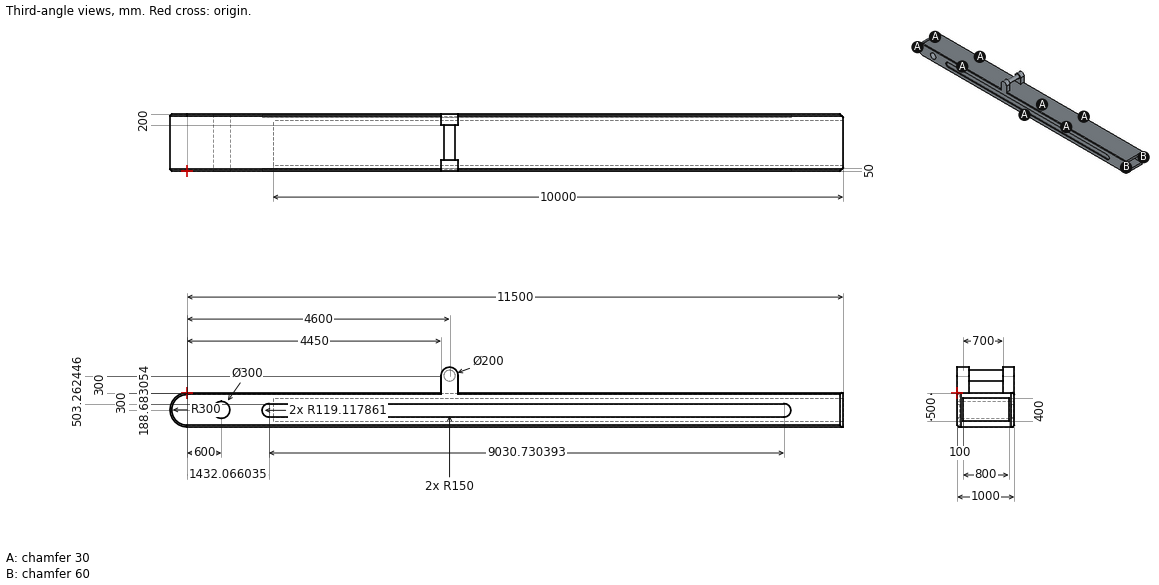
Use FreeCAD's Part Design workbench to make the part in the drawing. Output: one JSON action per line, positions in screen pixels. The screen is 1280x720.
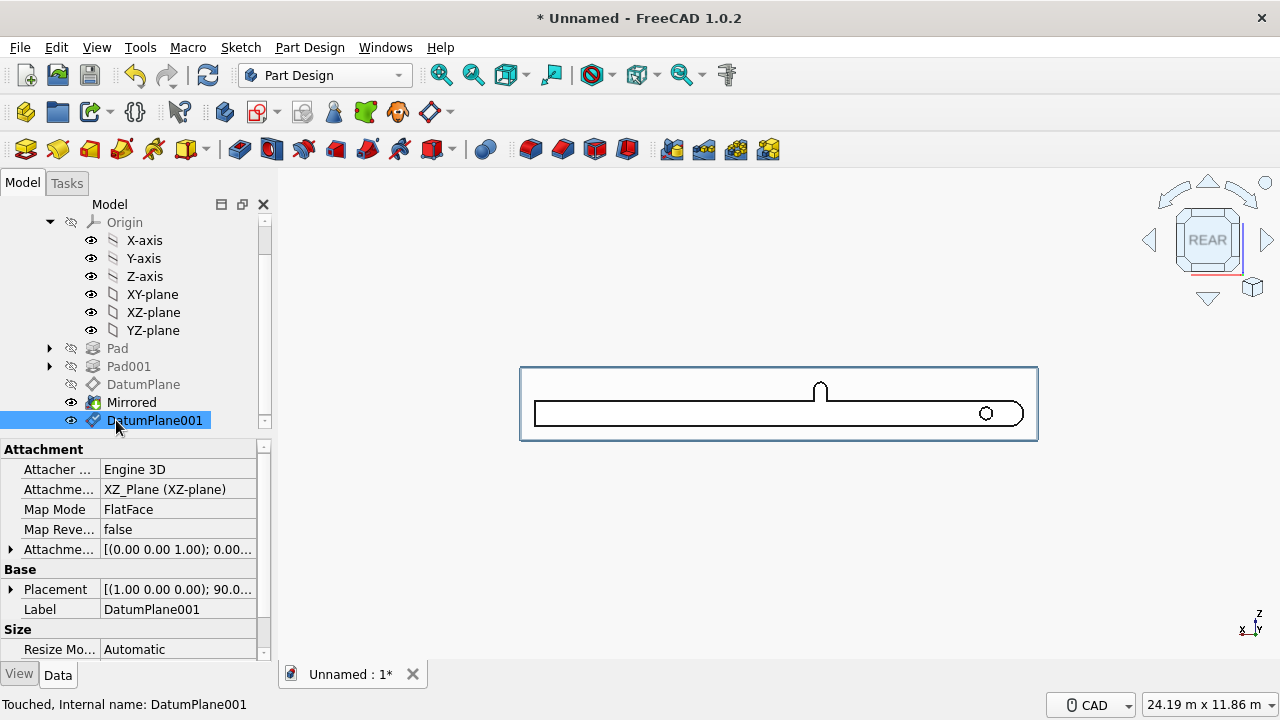
{"action": "left_click", "coordinate": [258, 112]}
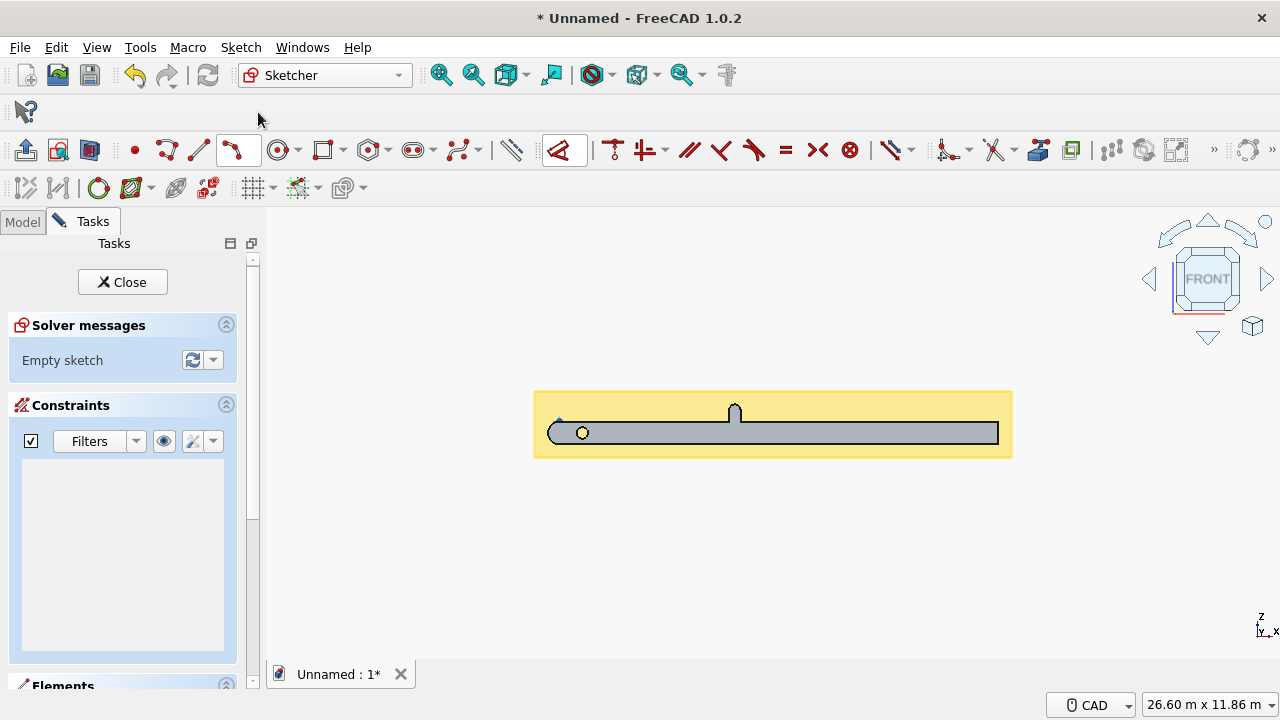
{"action": "left_click", "coordinate": [90, 150]}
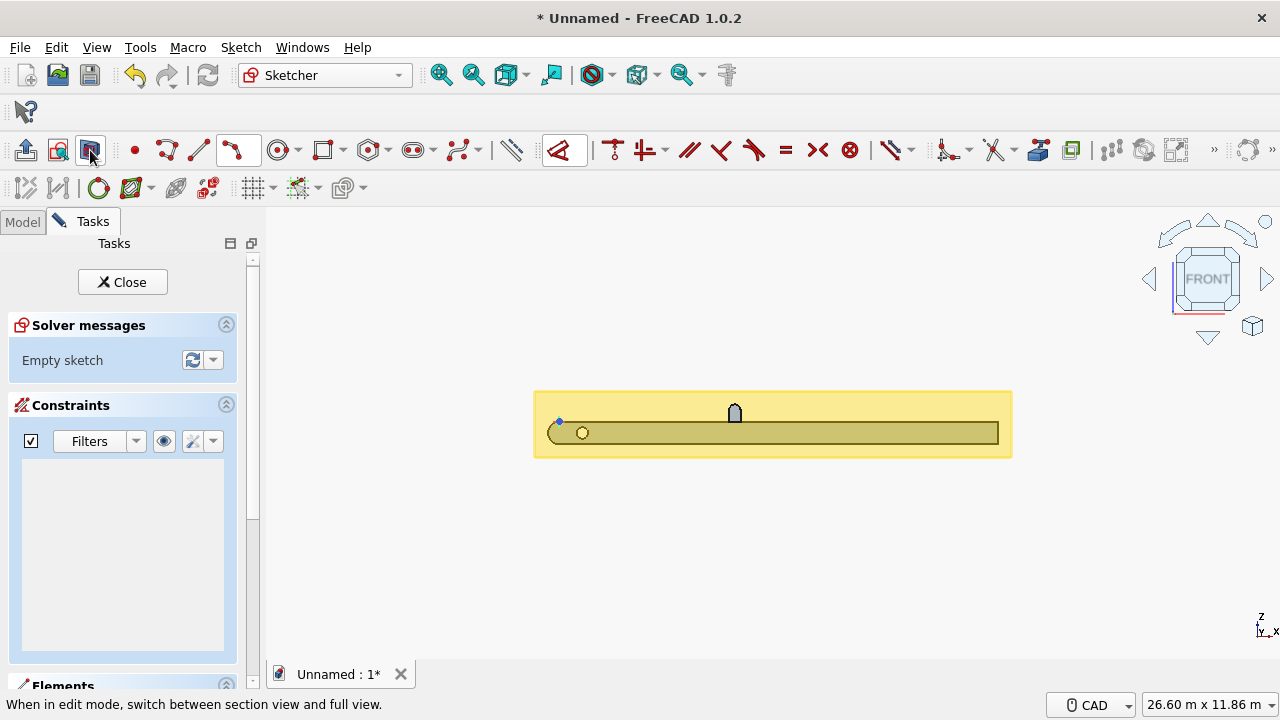
{"action": "scroll", "coordinate": [736, 409], "scroll_direction": "up", "scroll_amount": 15}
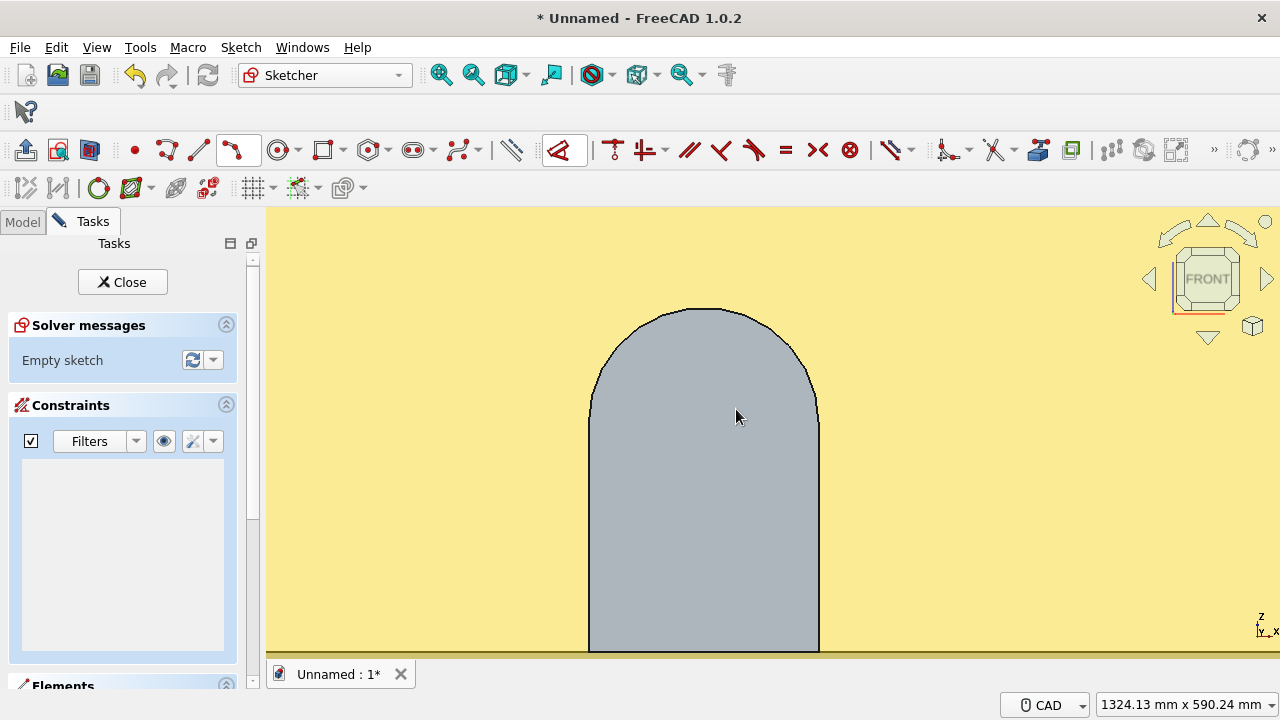
{"action": "scroll", "coordinate": [703, 410], "scroll_direction": "up", "scroll_amount": 3}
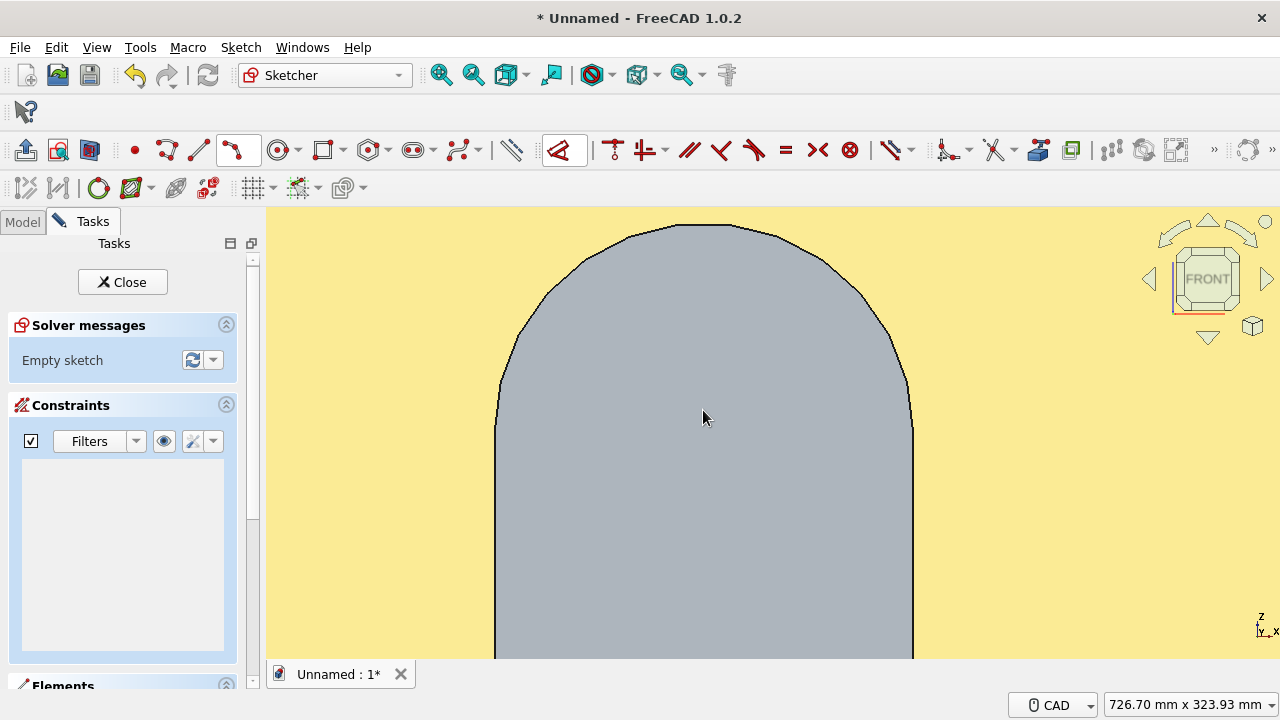
{"action": "left_click", "coordinate": [278, 150]}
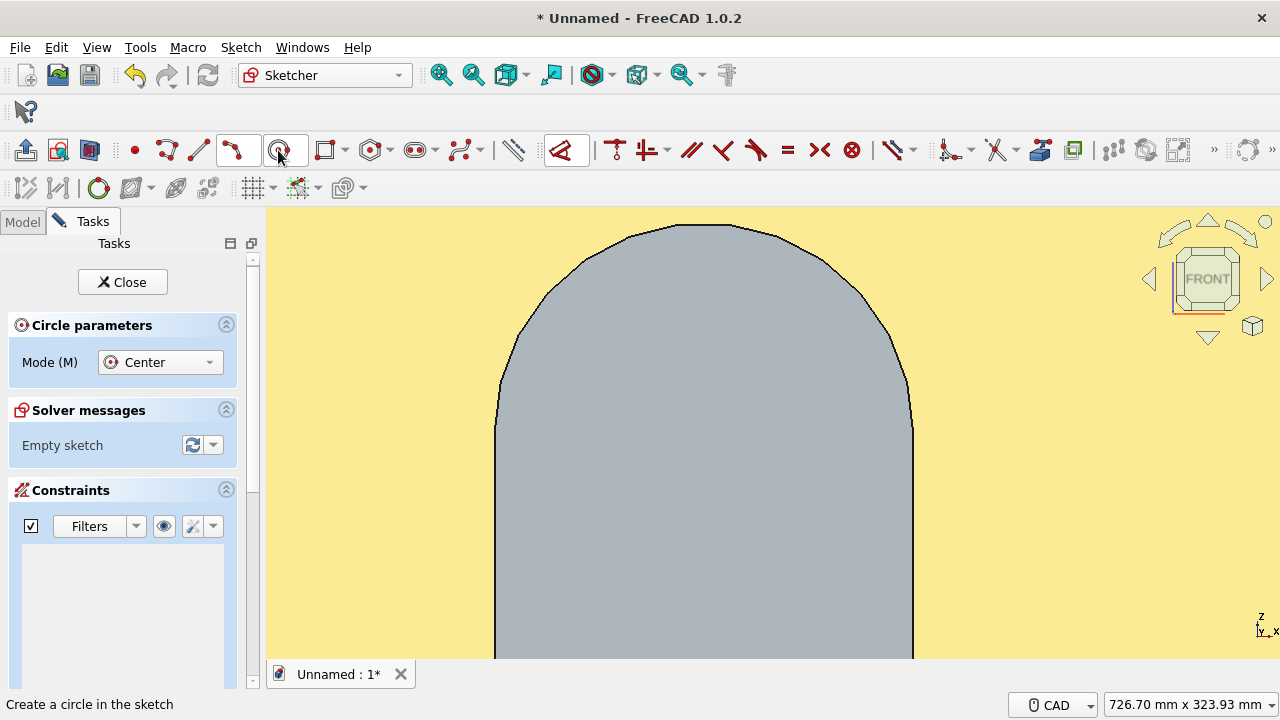
{"action": "left_click", "coordinate": [704, 432]}
{"action": "left_click", "coordinate": [803, 334]}
{"action": "key", "text": "Escape"}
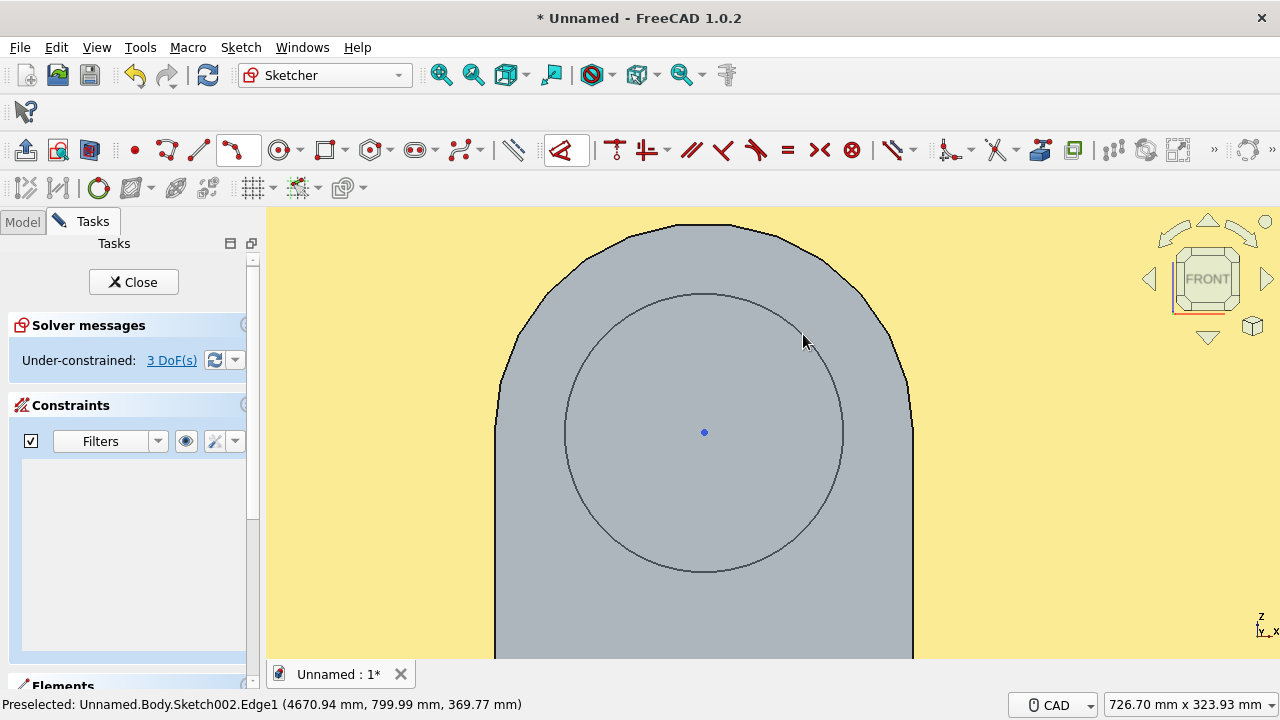
{"action": "left_click", "coordinate": [802, 334]}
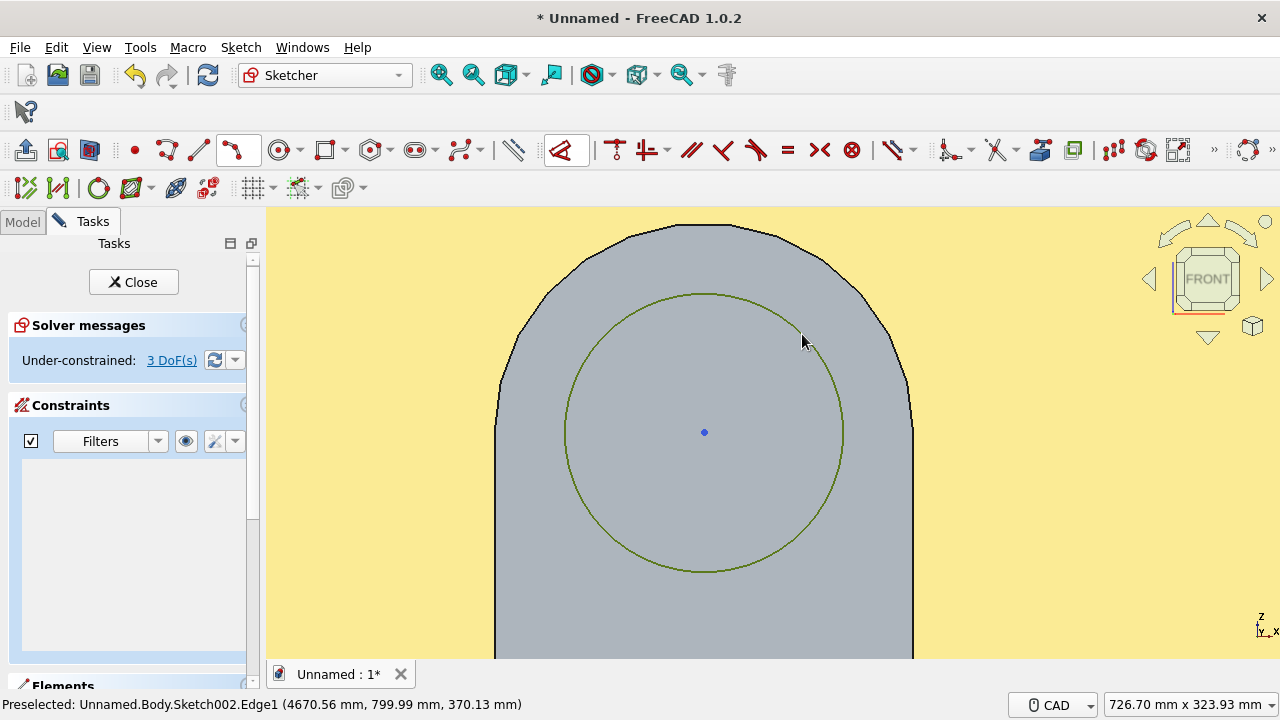
{"action": "left_click", "coordinate": [584, 150]}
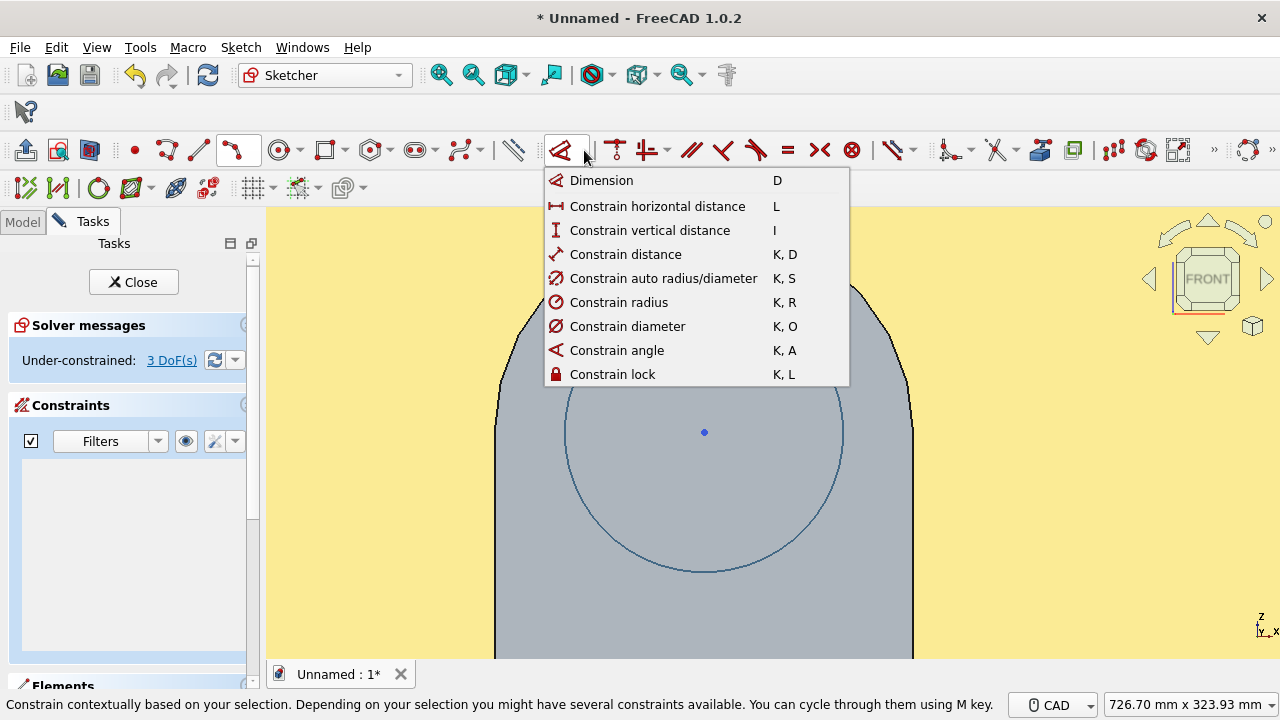
{"action": "left_click", "coordinate": [697, 326]}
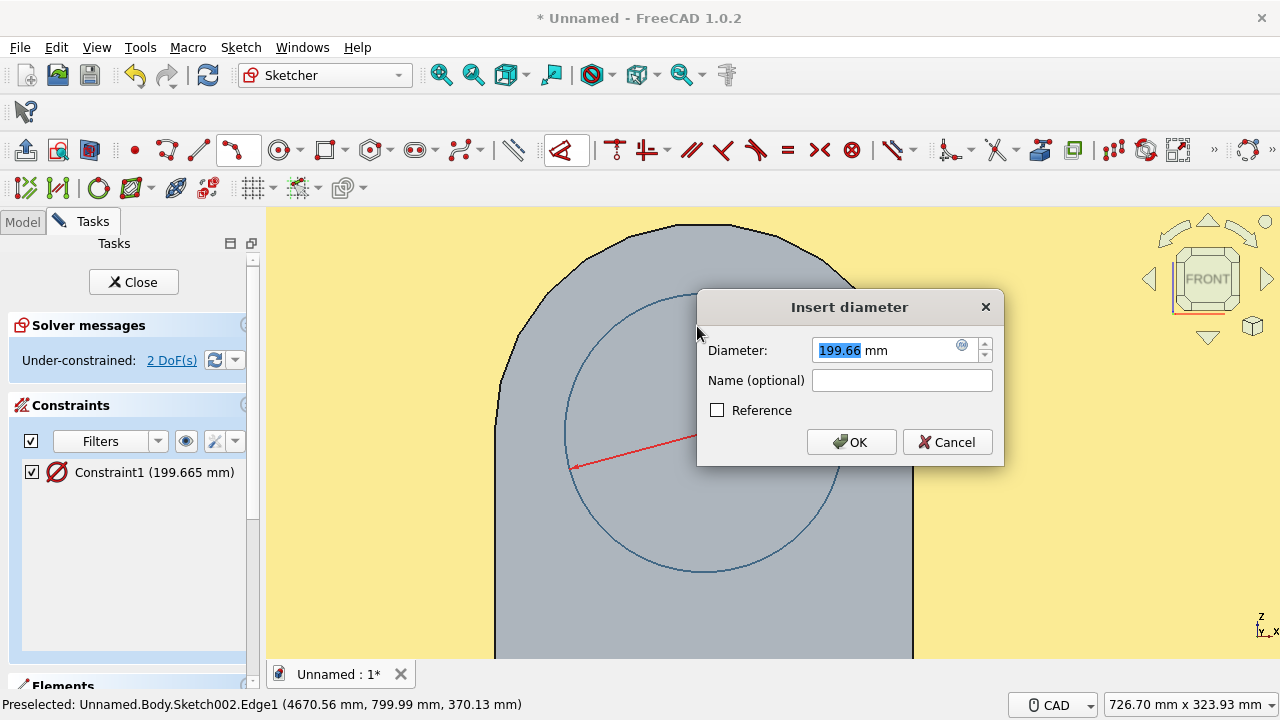
{"action": "type", "text": "200"}
{"action": "key", "text": "Return"}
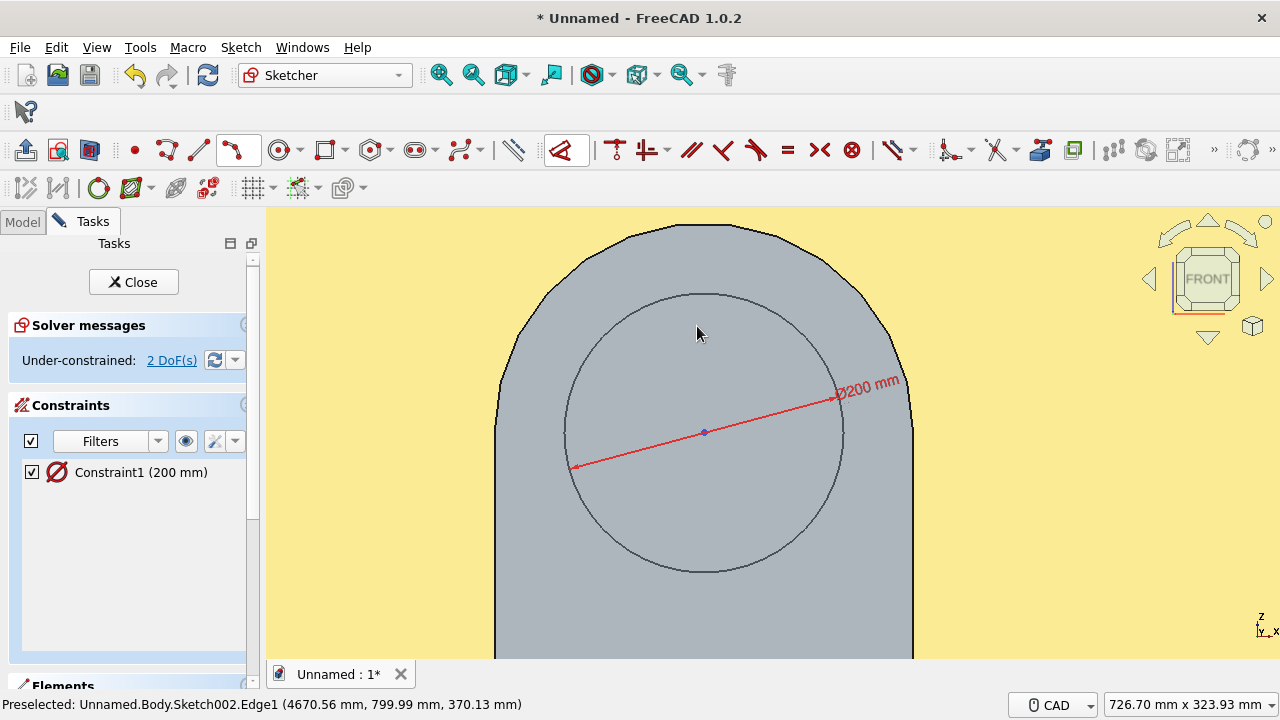
{"action": "left_click", "coordinate": [704, 433]}